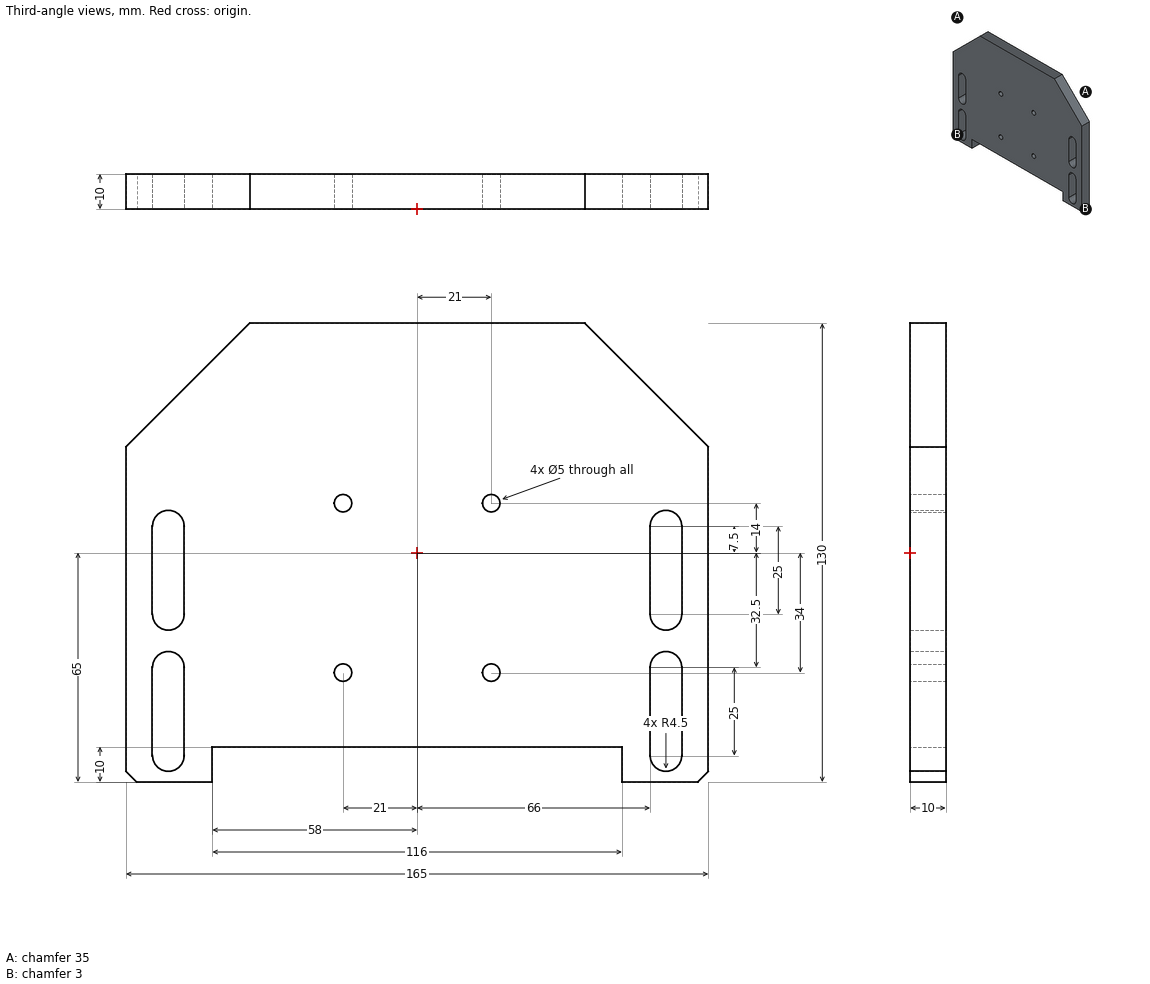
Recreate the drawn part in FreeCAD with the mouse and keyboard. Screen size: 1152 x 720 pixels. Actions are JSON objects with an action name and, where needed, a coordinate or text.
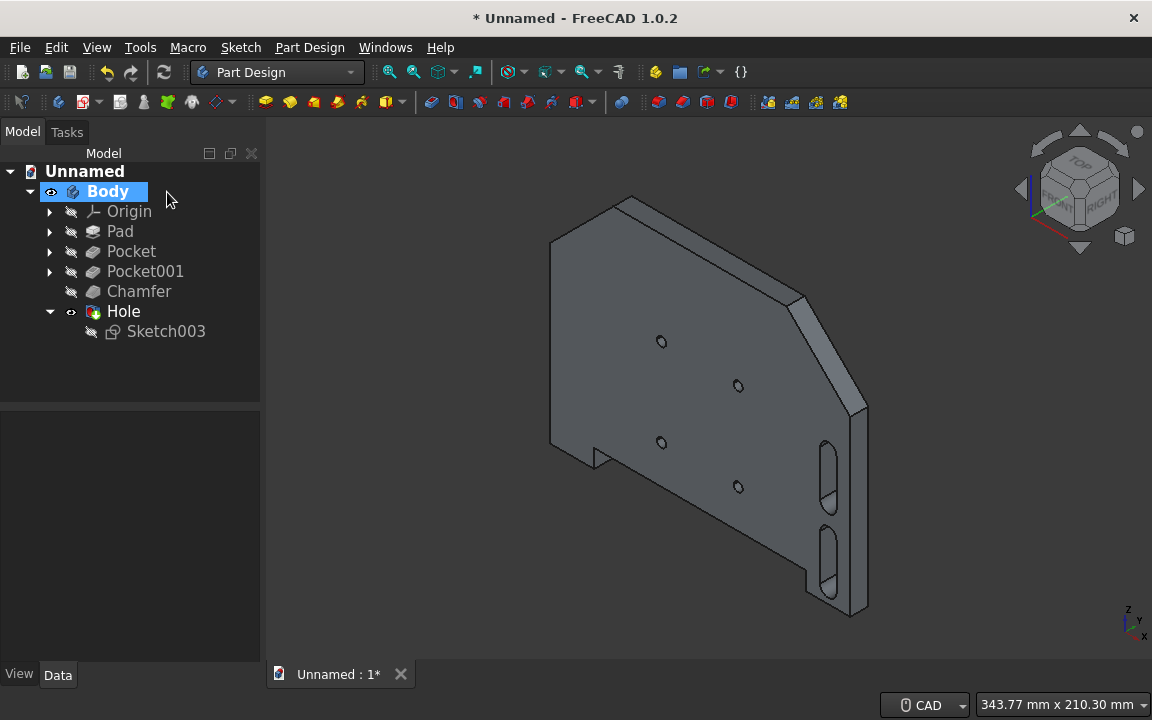
{"action": "key", "text": "2"}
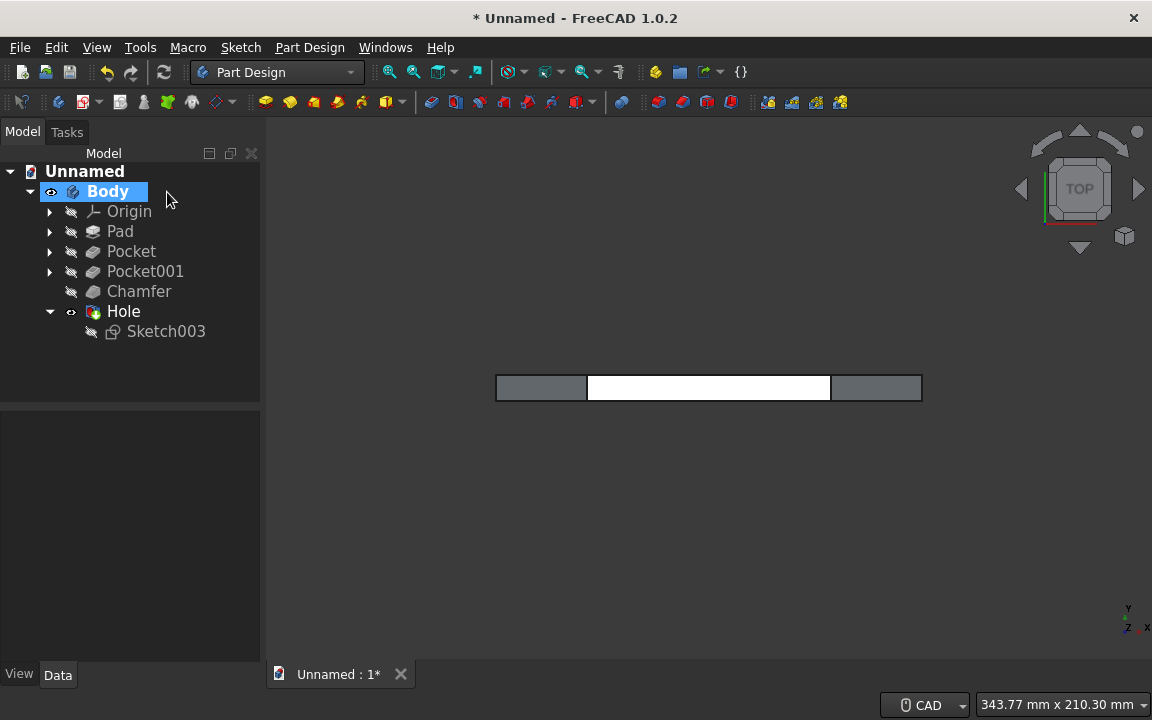
{"action": "key", "text": "1"}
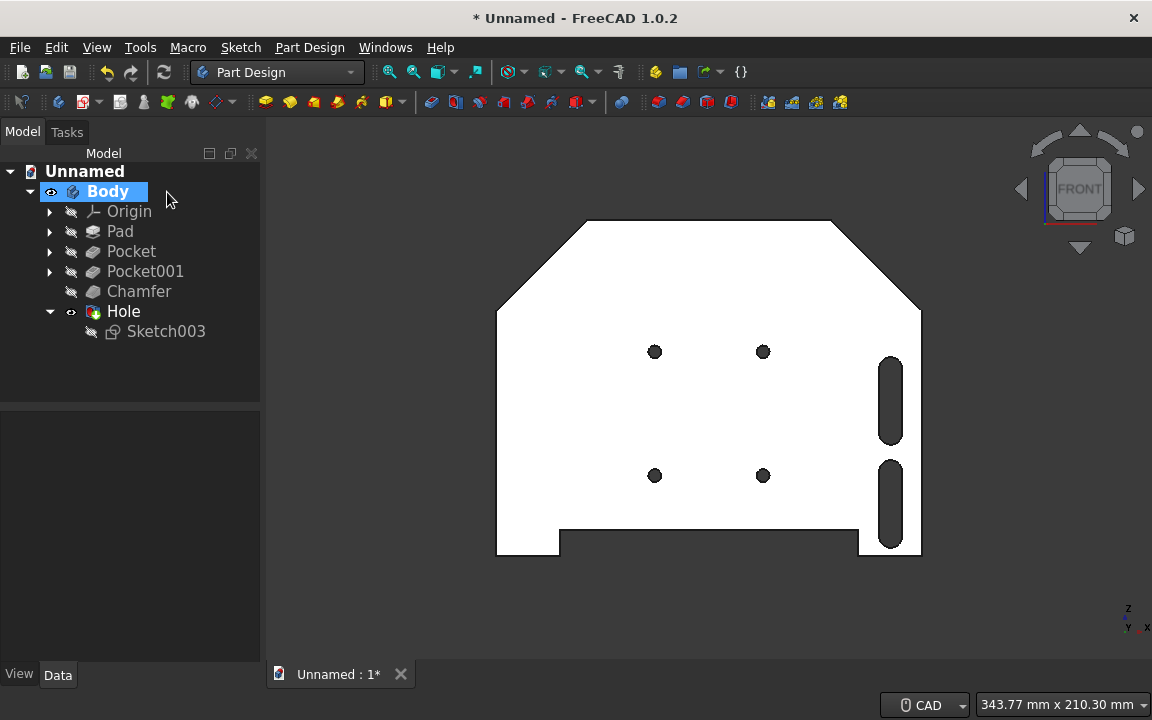
{"action": "key", "text": "3"}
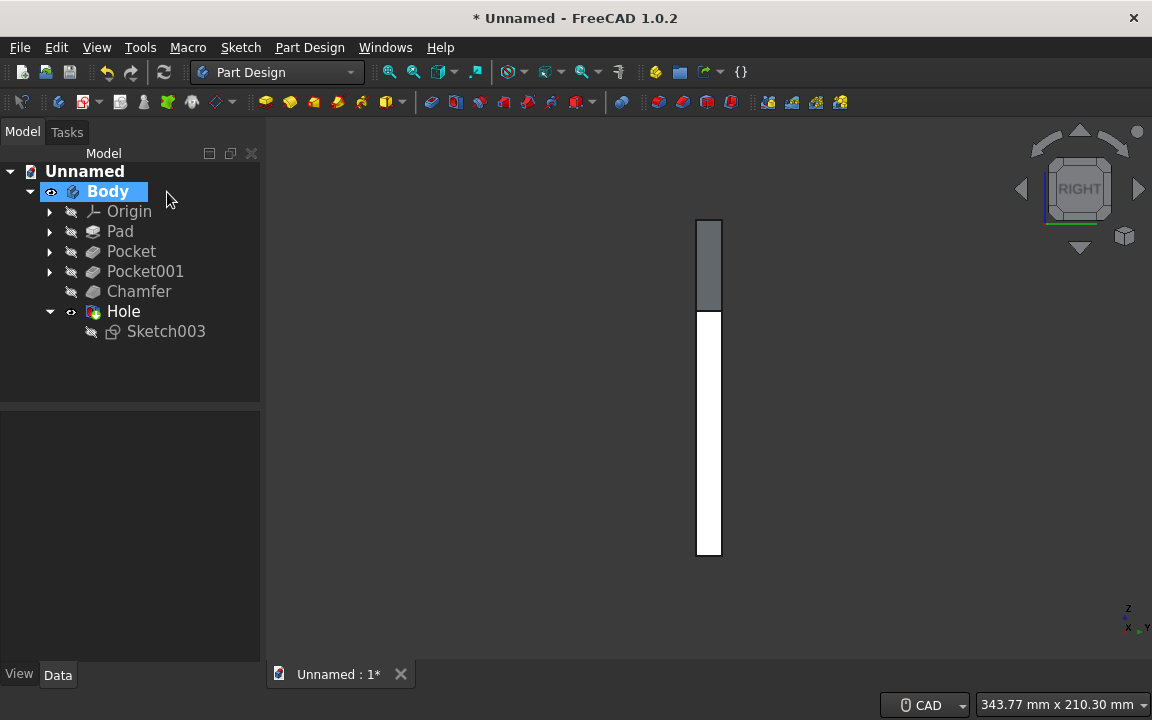
{"action": "left_click", "coordinate": [709, 555]}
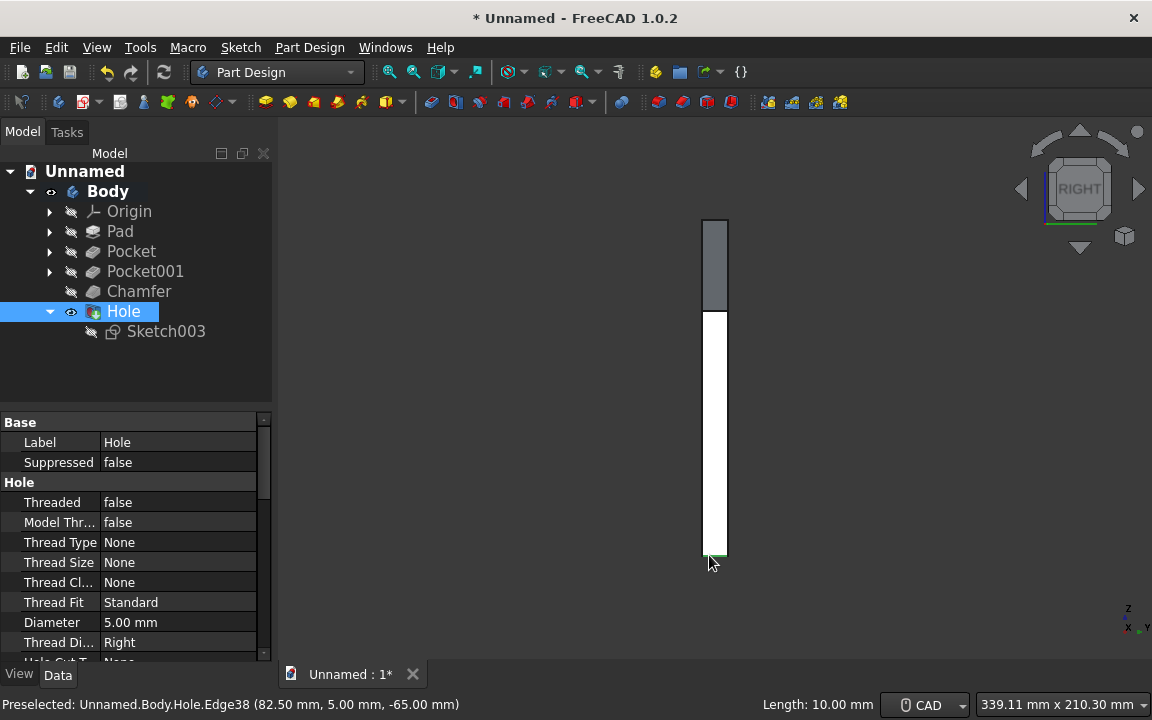
{"action": "key", "text": "5"}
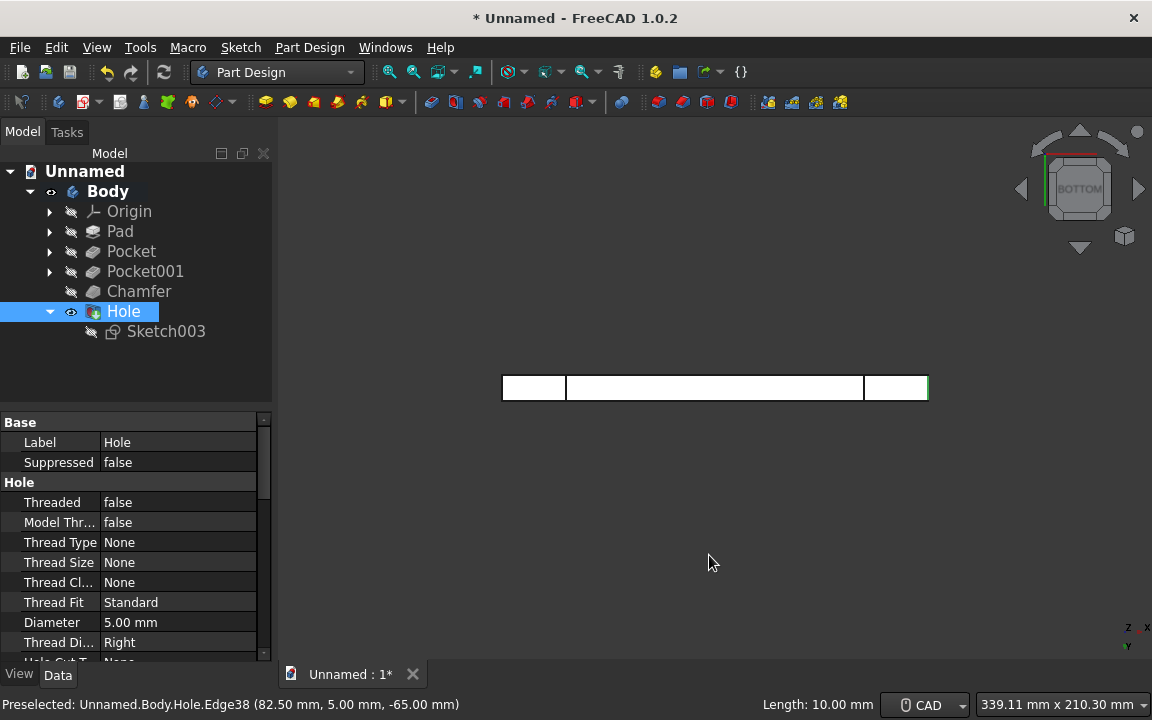
{"action": "left_click", "coordinate": [502, 387], "text": "ctrl"}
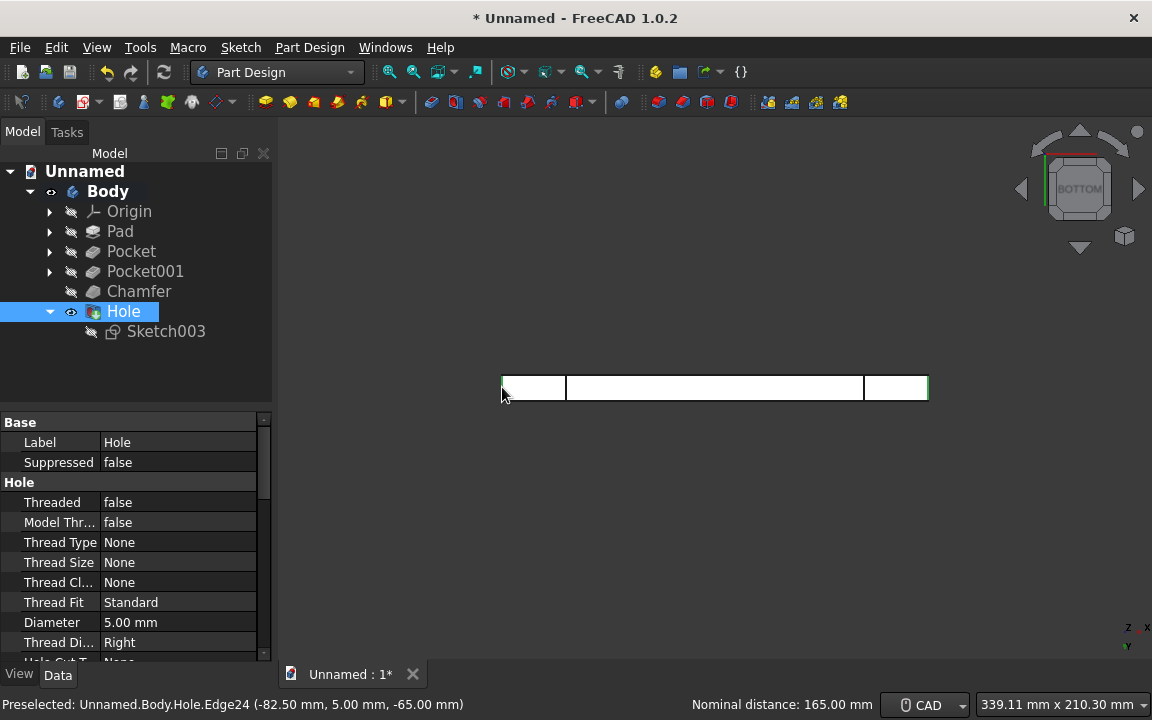
{"action": "left_click", "coordinate": [684, 102]}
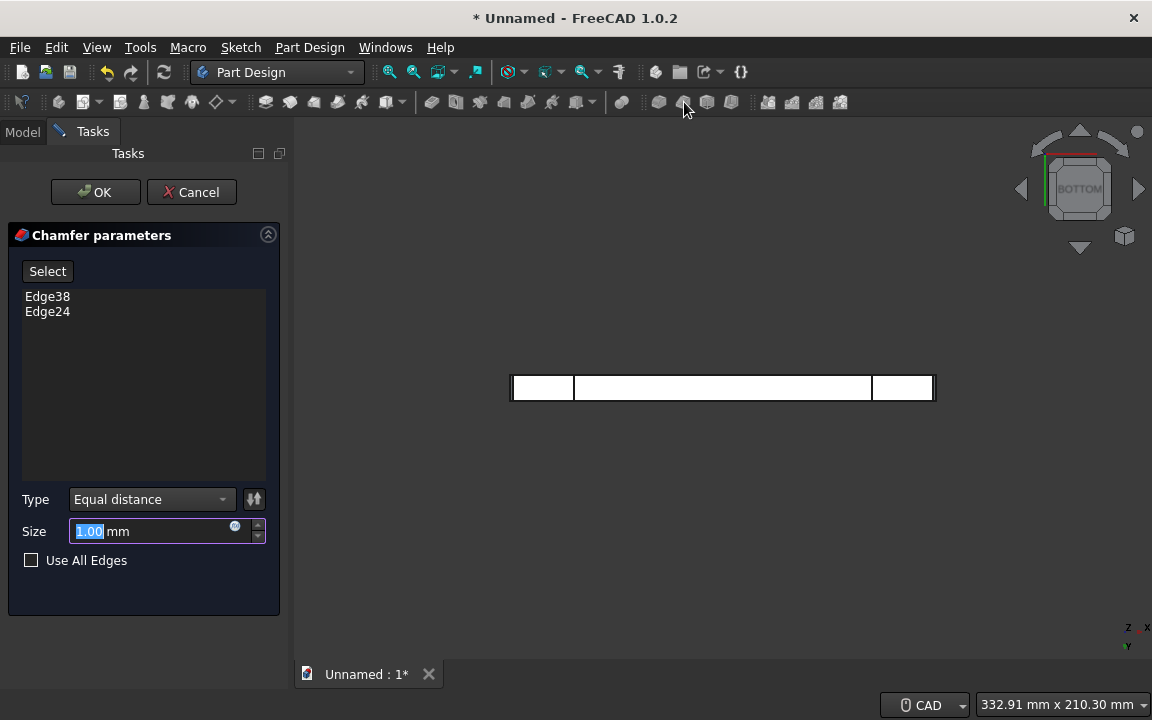
{"action": "type", "text": "3"}
{"action": "key", "text": "Tab"}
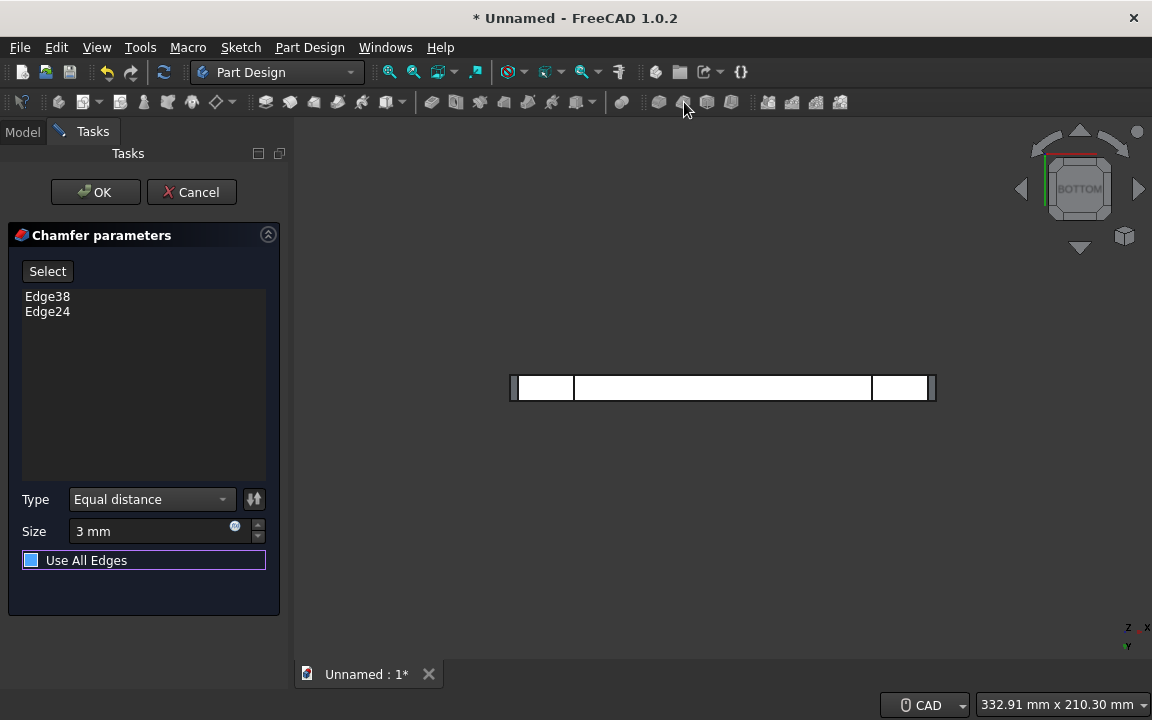
{"action": "left_click", "coordinate": [96, 192]}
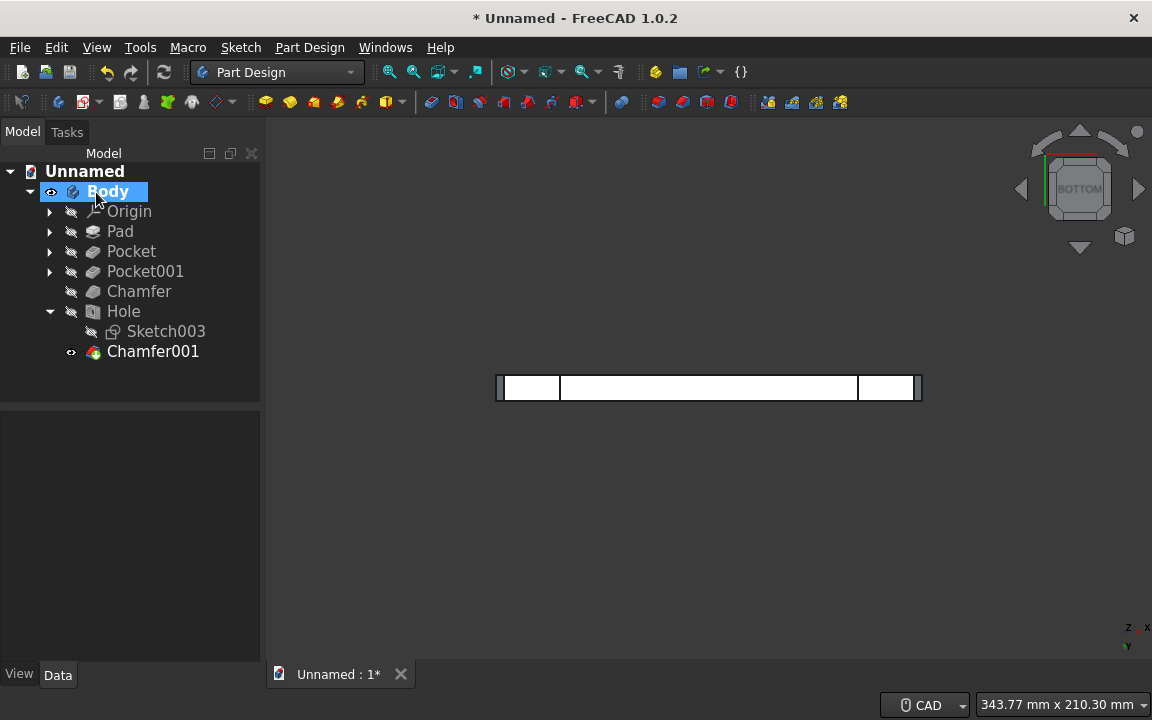
{"action": "left_click", "coordinate": [116, 272]}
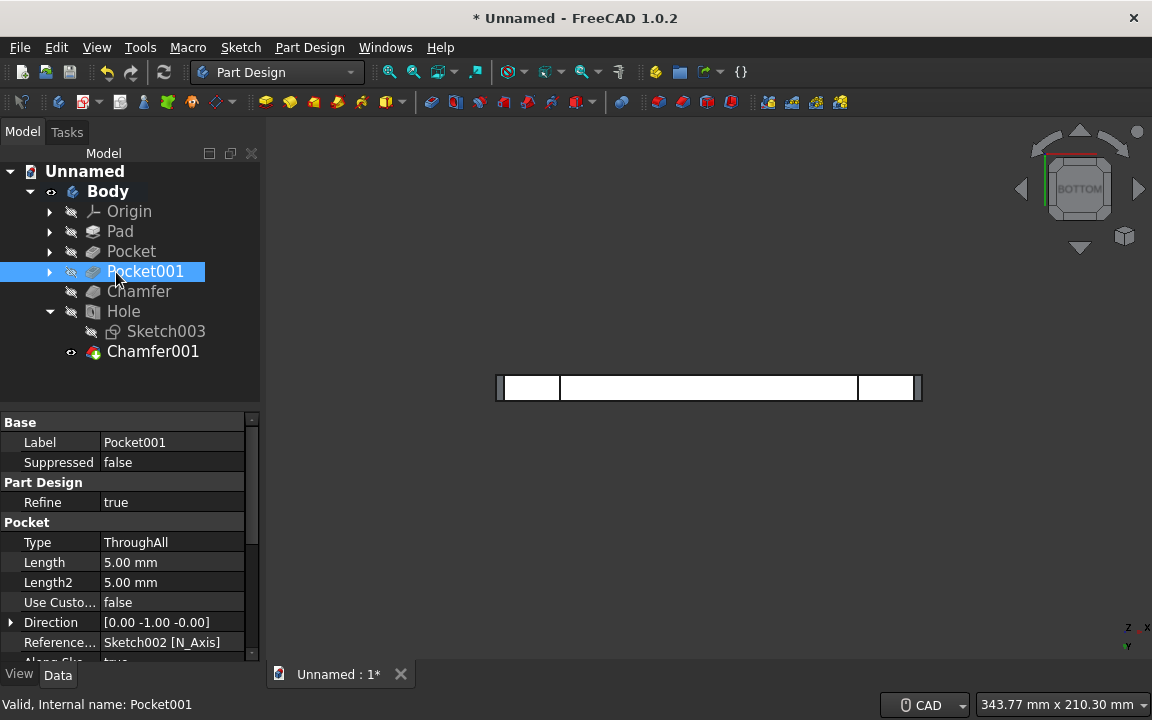
{"action": "left_click", "coordinate": [768, 102]}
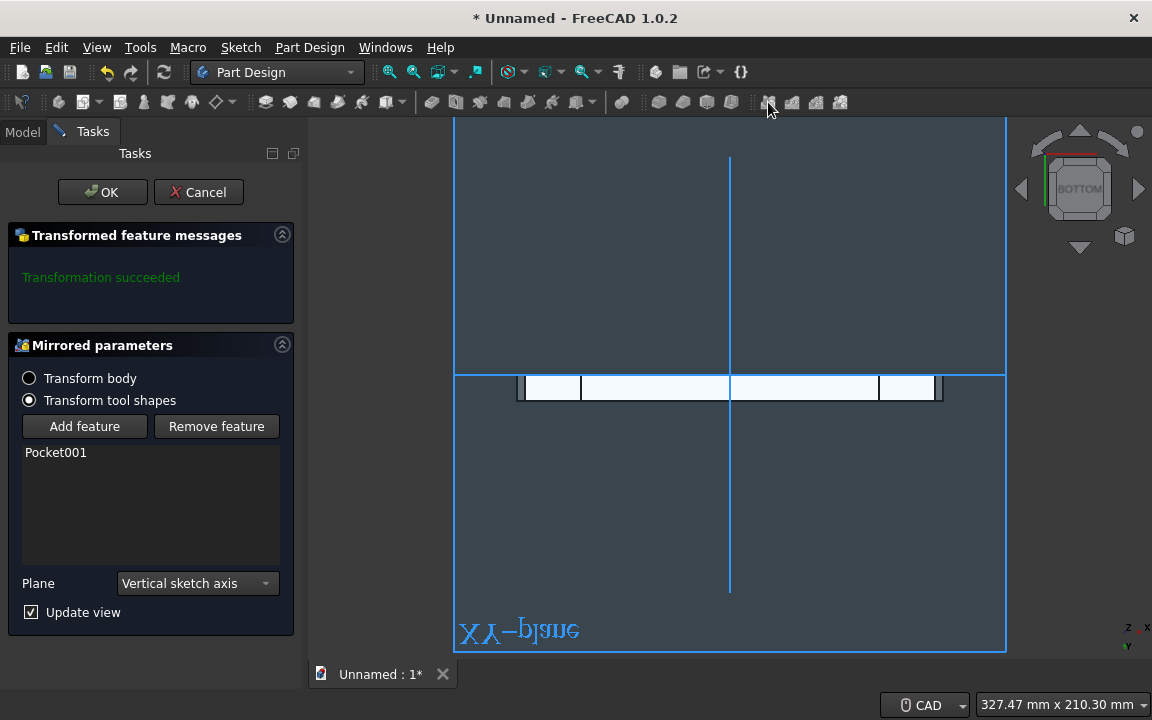
{"action": "left_click", "coordinate": [198, 584]}